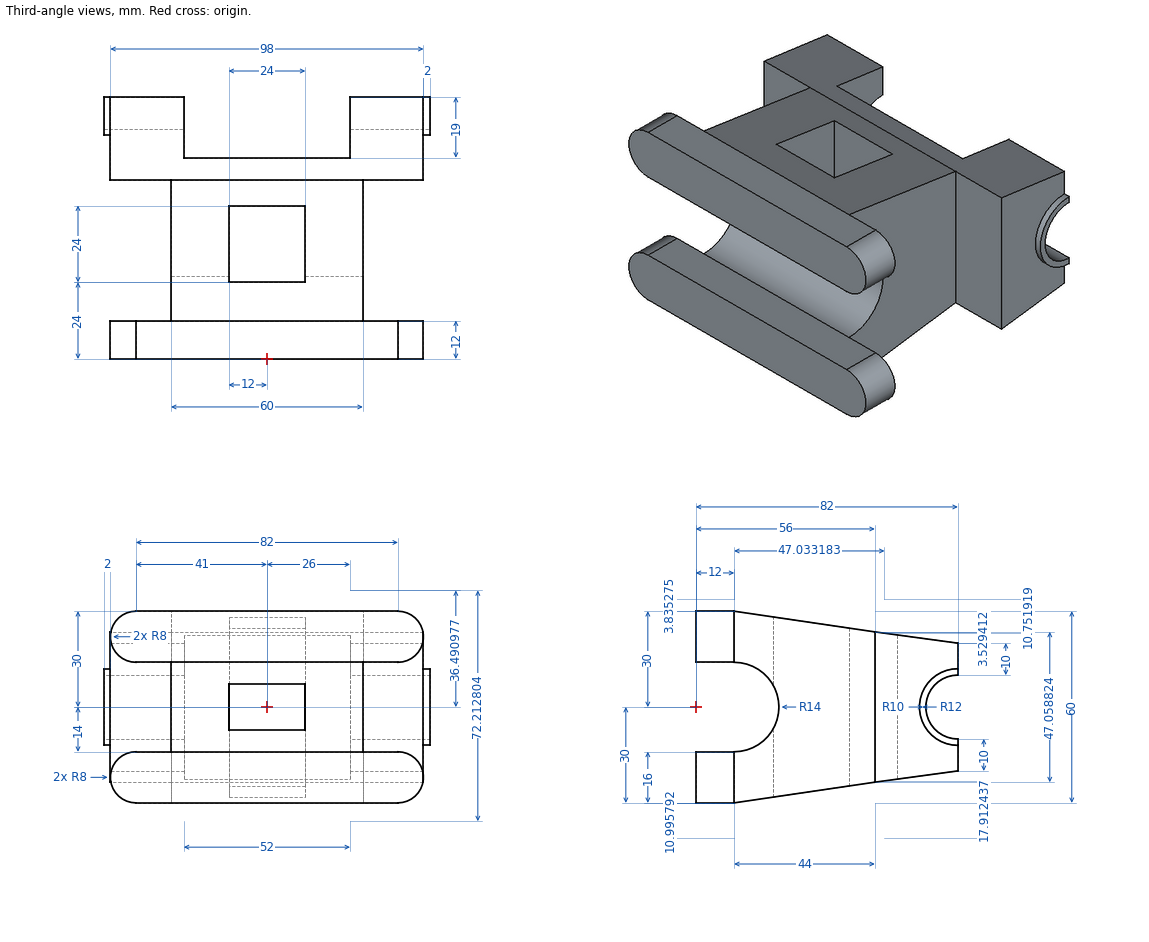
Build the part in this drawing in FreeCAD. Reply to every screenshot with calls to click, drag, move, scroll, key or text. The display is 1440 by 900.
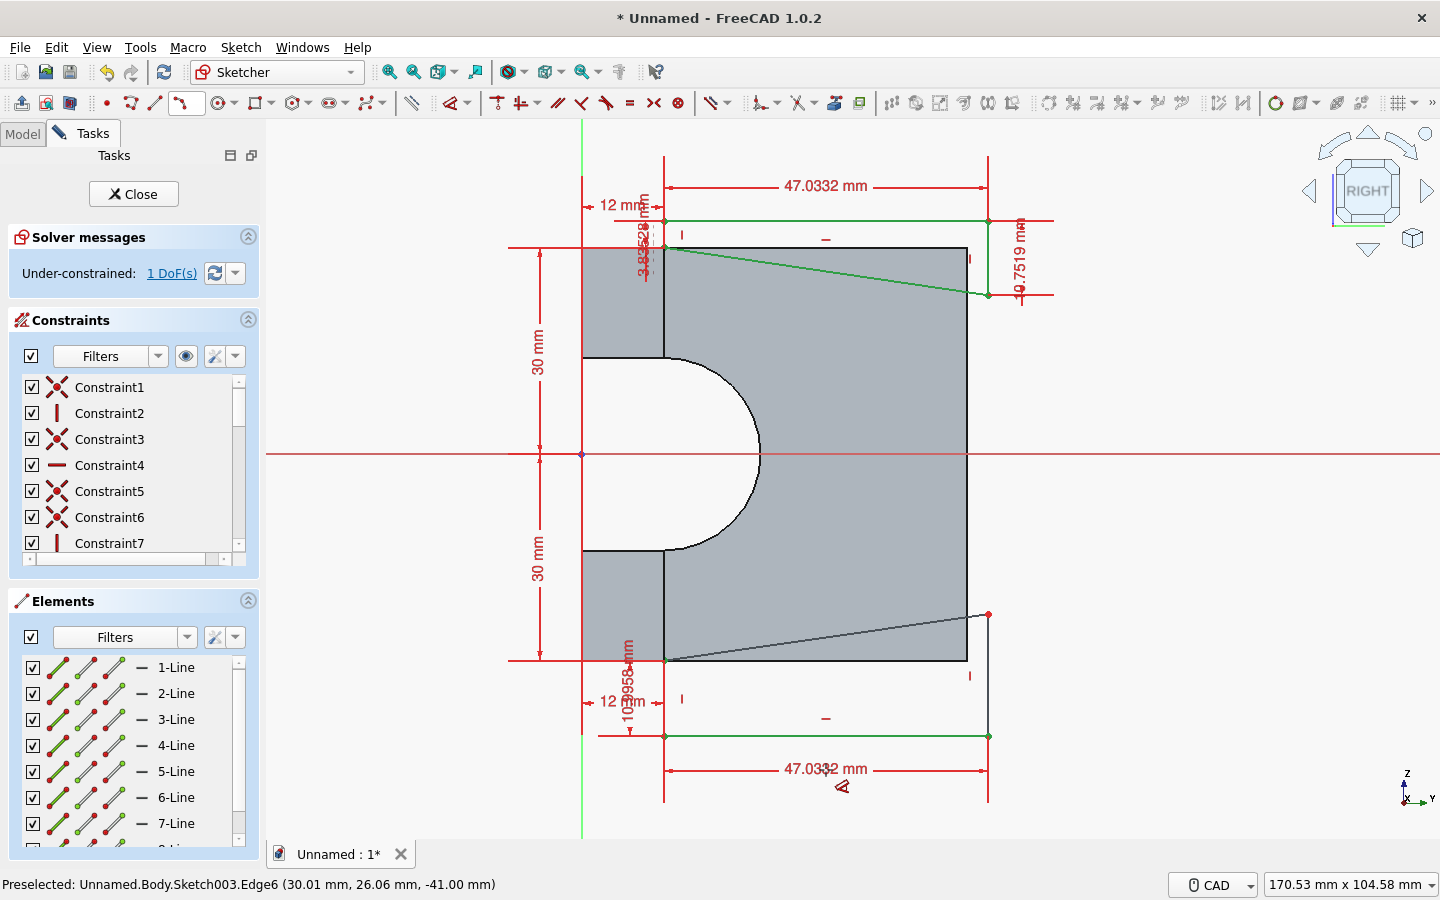
click(988, 700)
click(1022, 675)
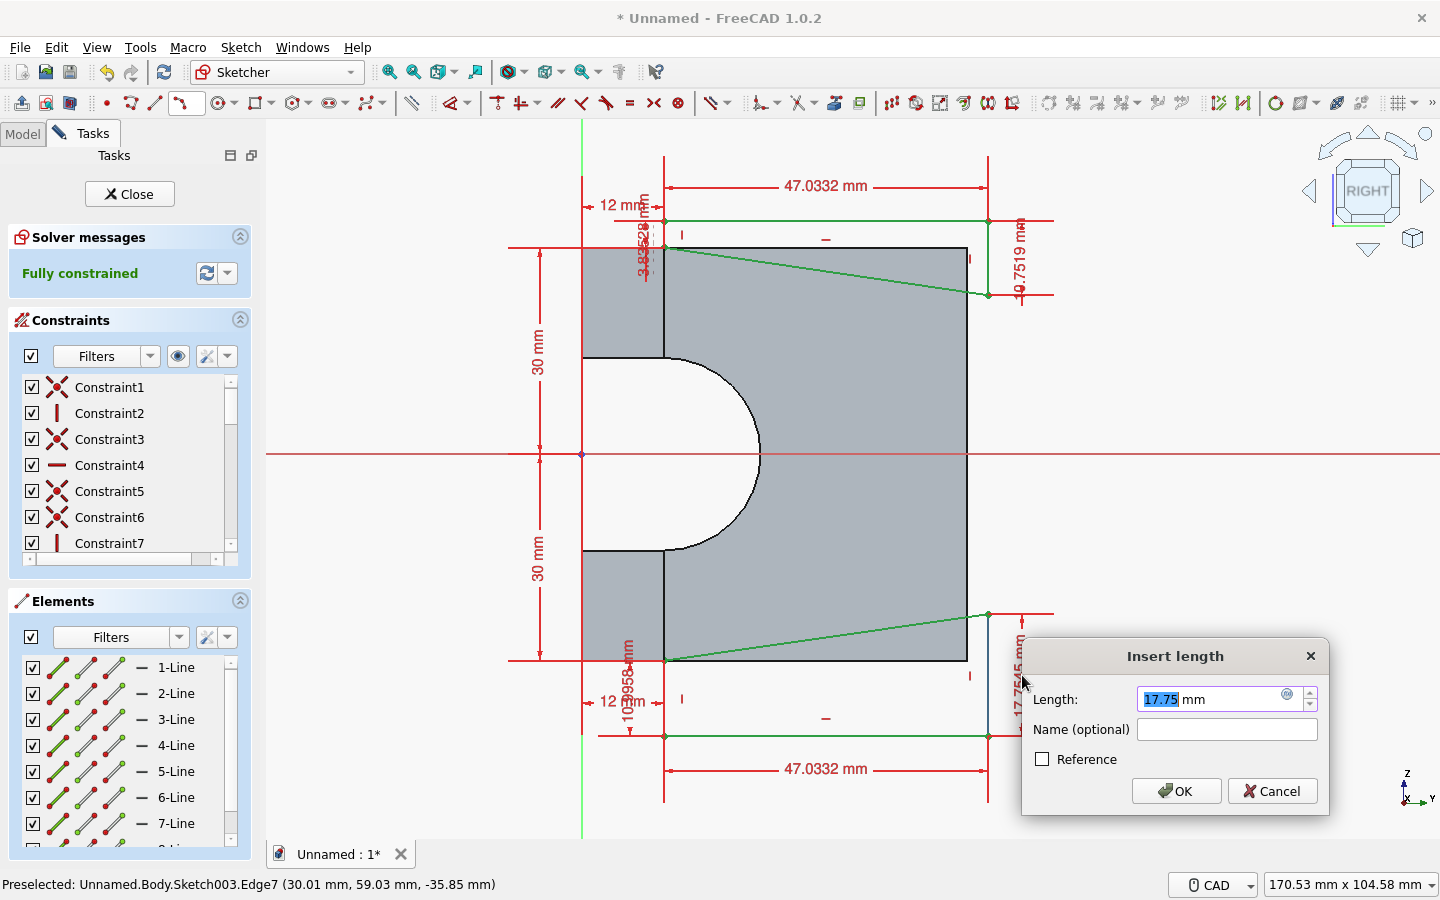
text(17.912437)
key(Return)
key(Escape)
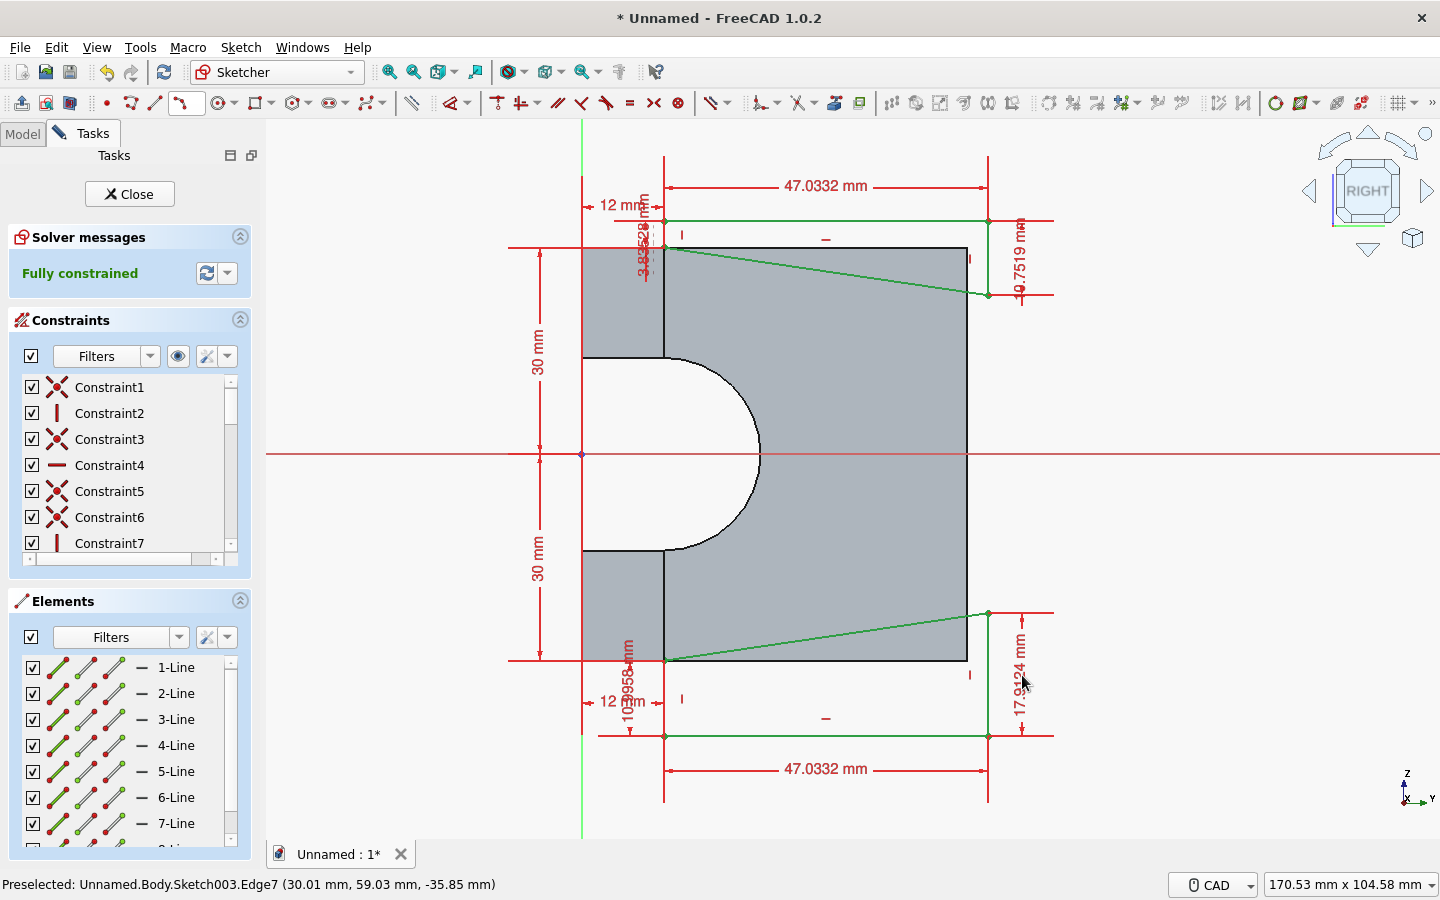
click(130, 194)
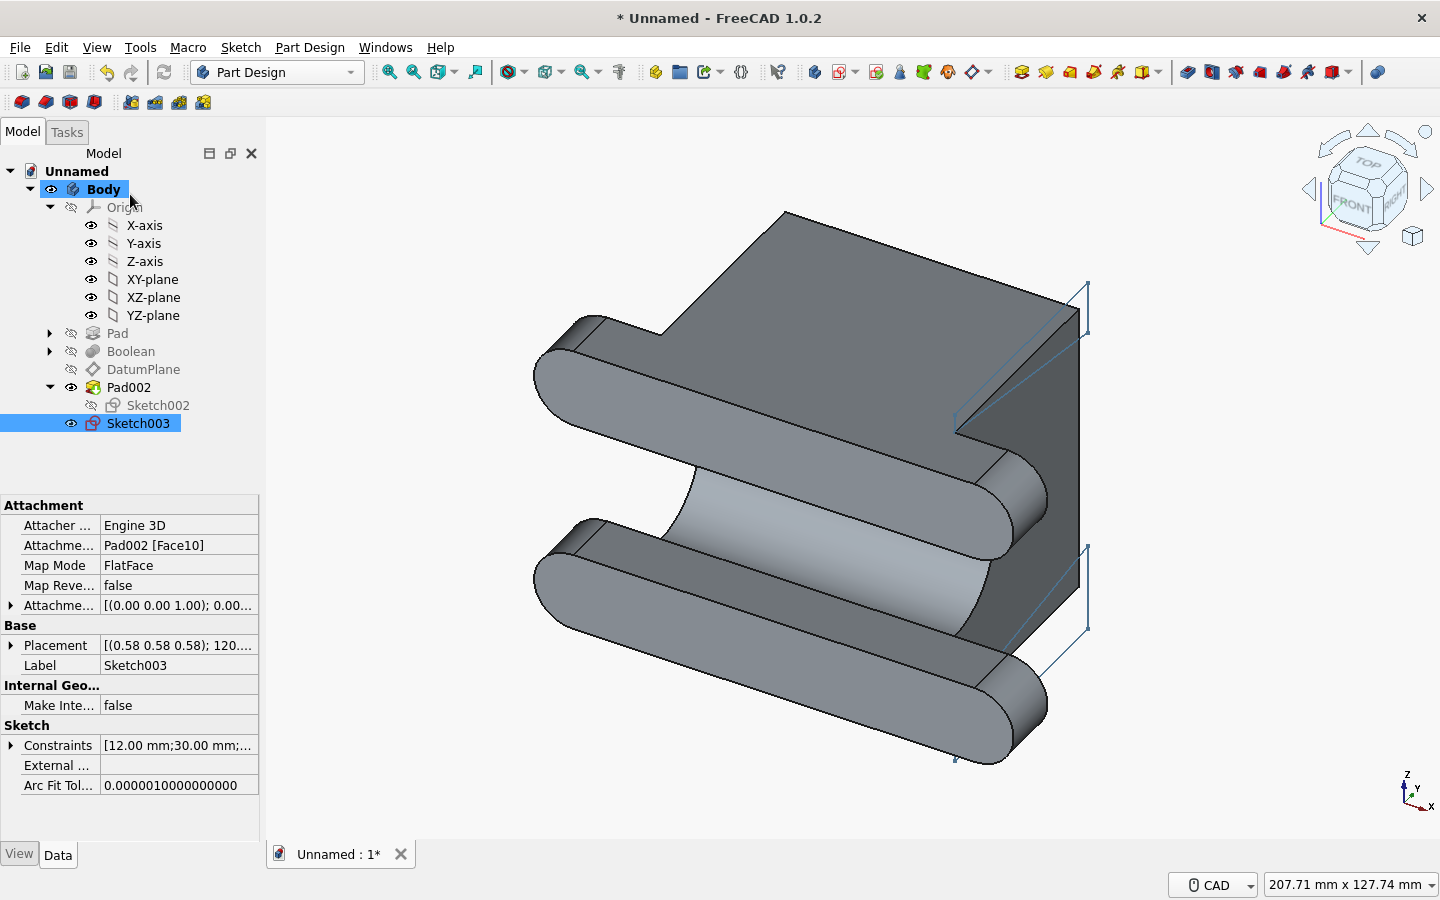
click(1188, 72)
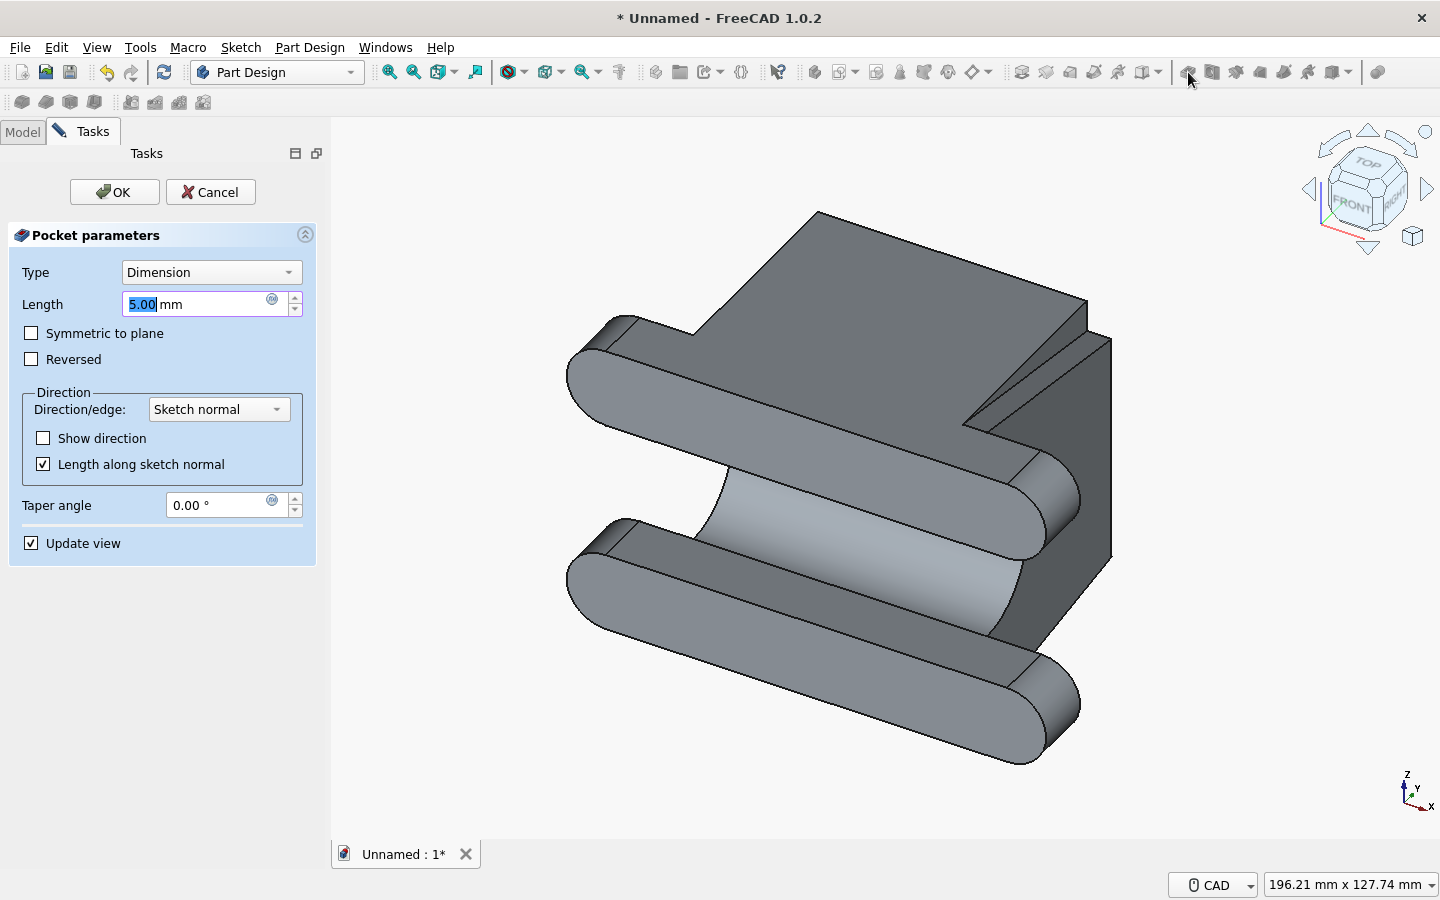
text(60)
key(Tab)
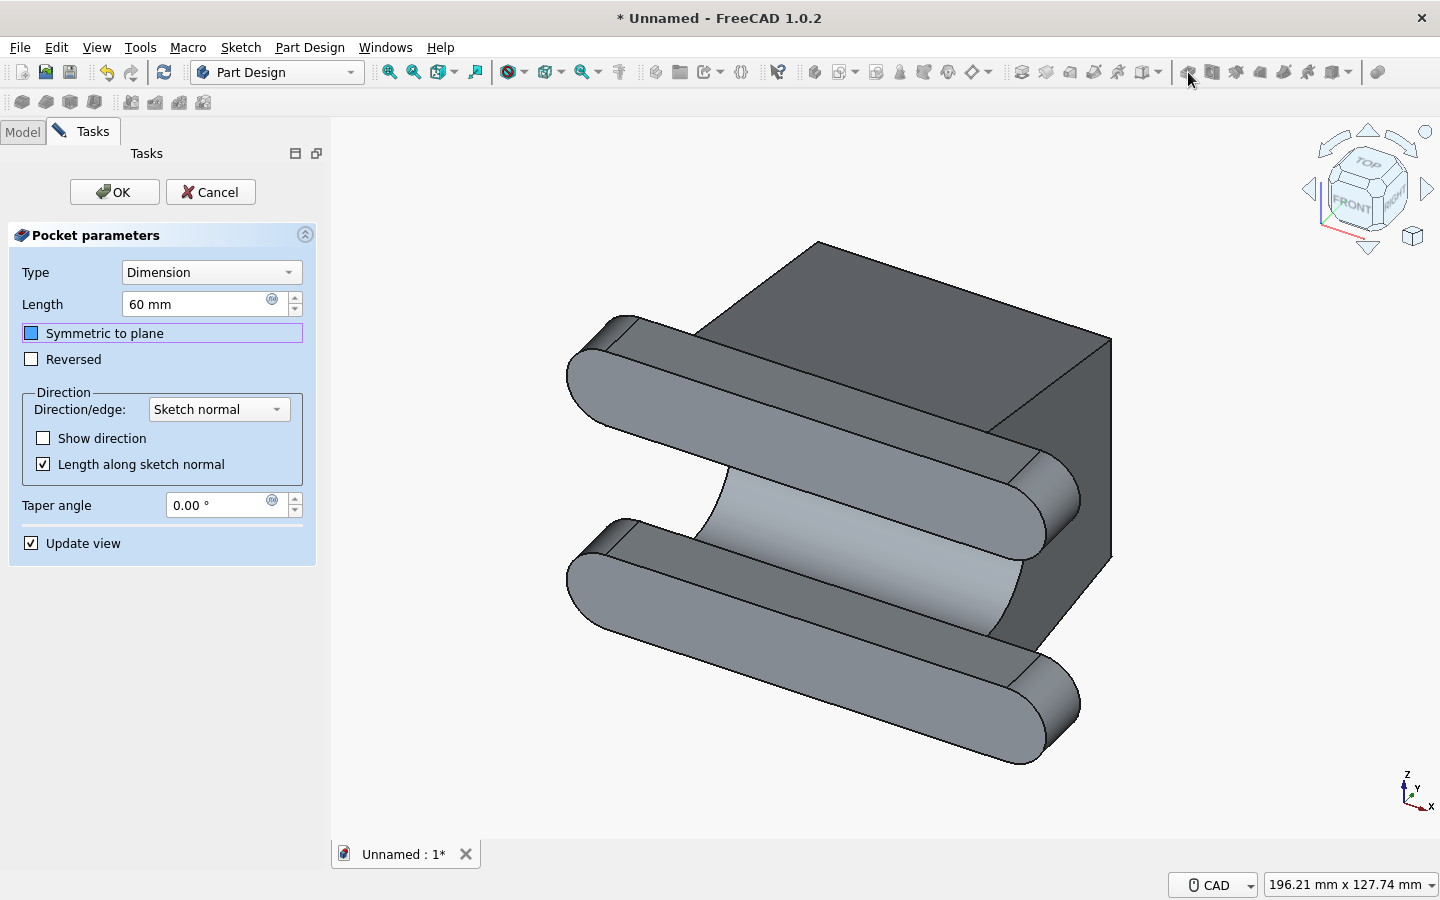
click(115, 192)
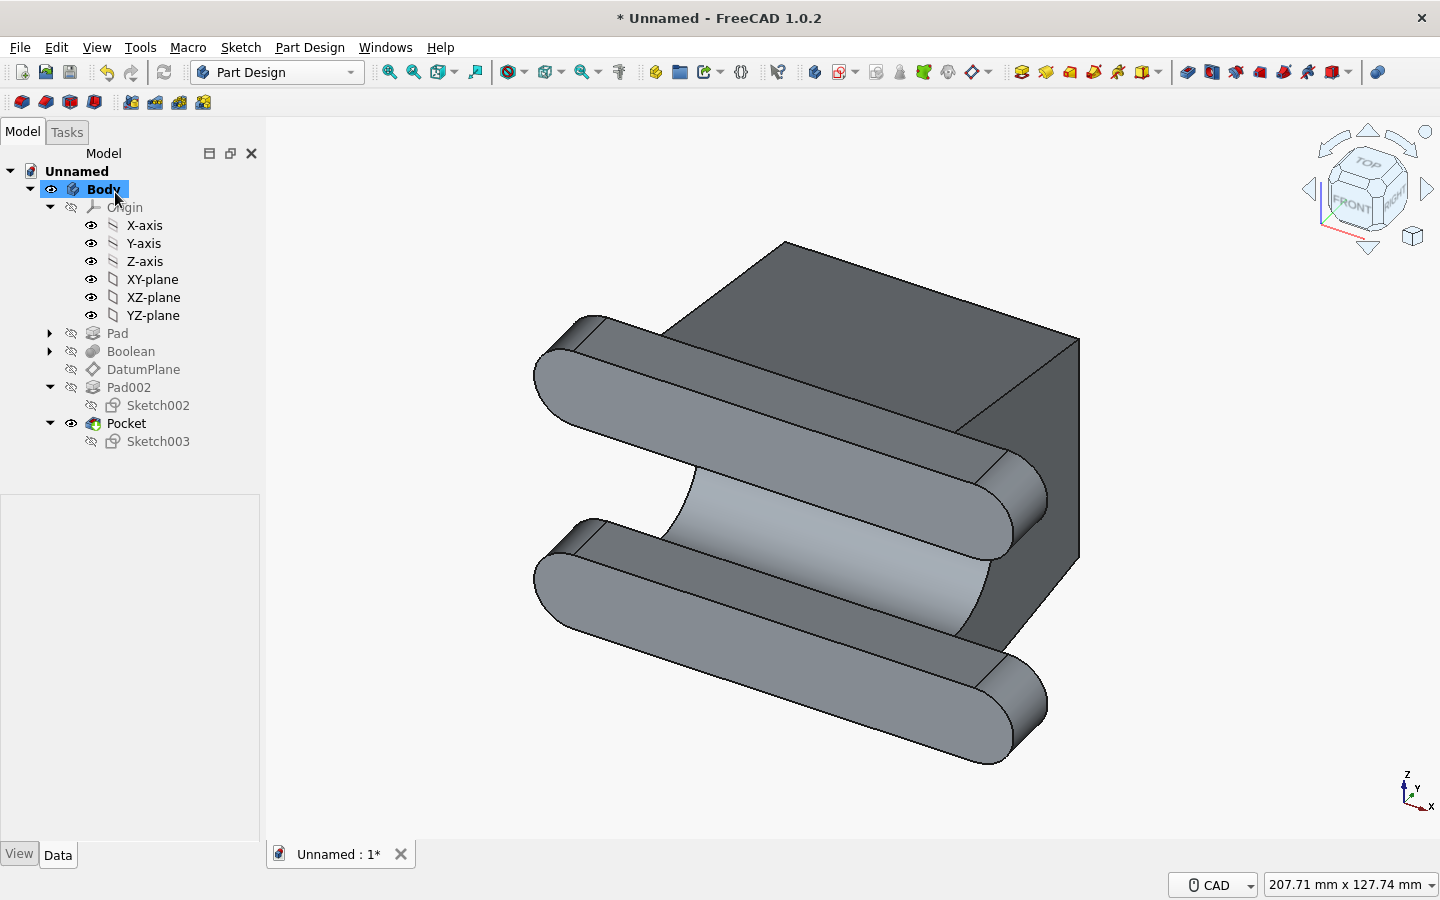
click(136, 315)